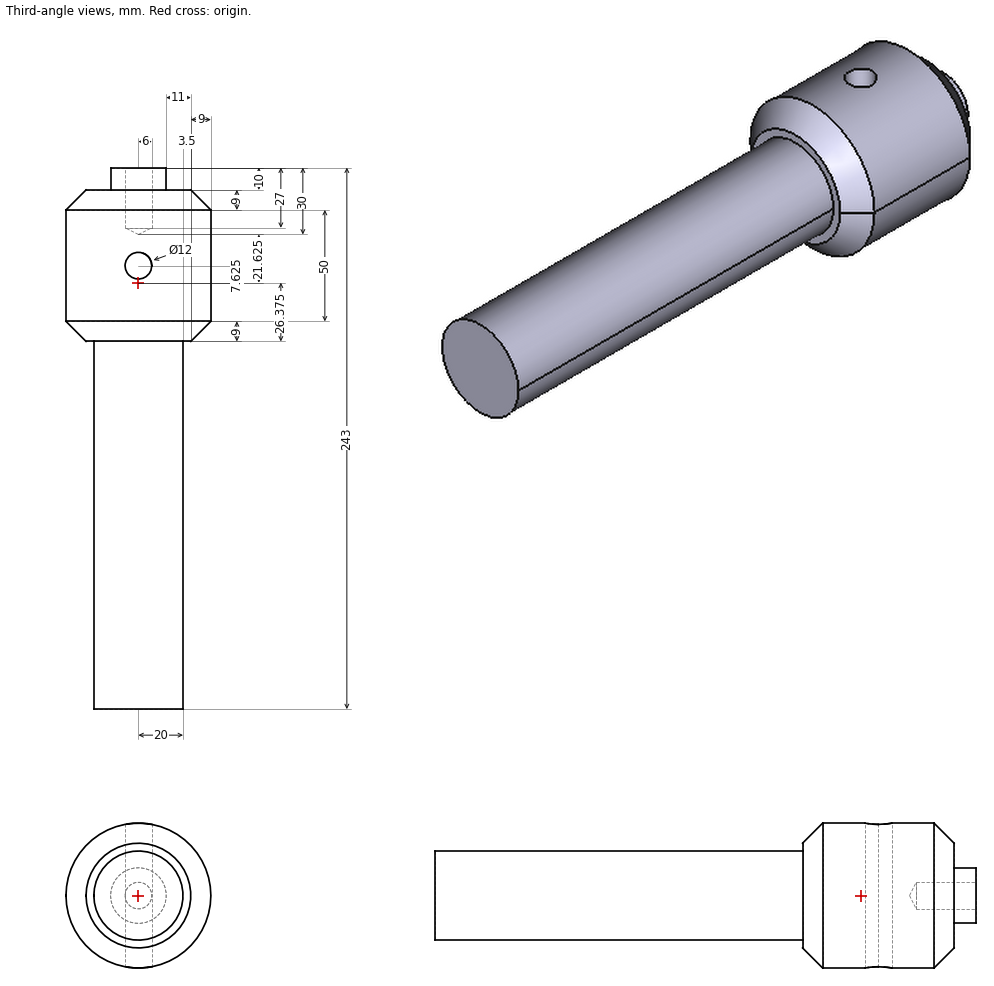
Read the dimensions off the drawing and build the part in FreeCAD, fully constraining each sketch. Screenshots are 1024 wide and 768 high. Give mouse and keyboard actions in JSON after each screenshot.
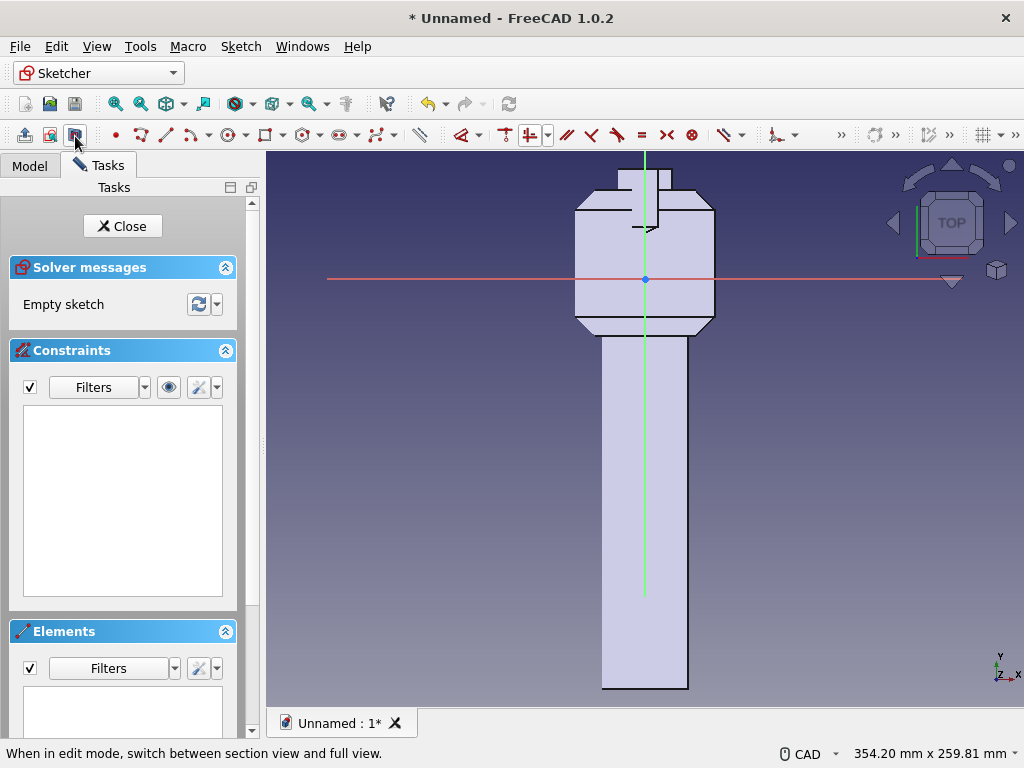
{"action": "scroll", "coordinate": [652, 249], "scroll_direction": "up", "scroll_amount": 12}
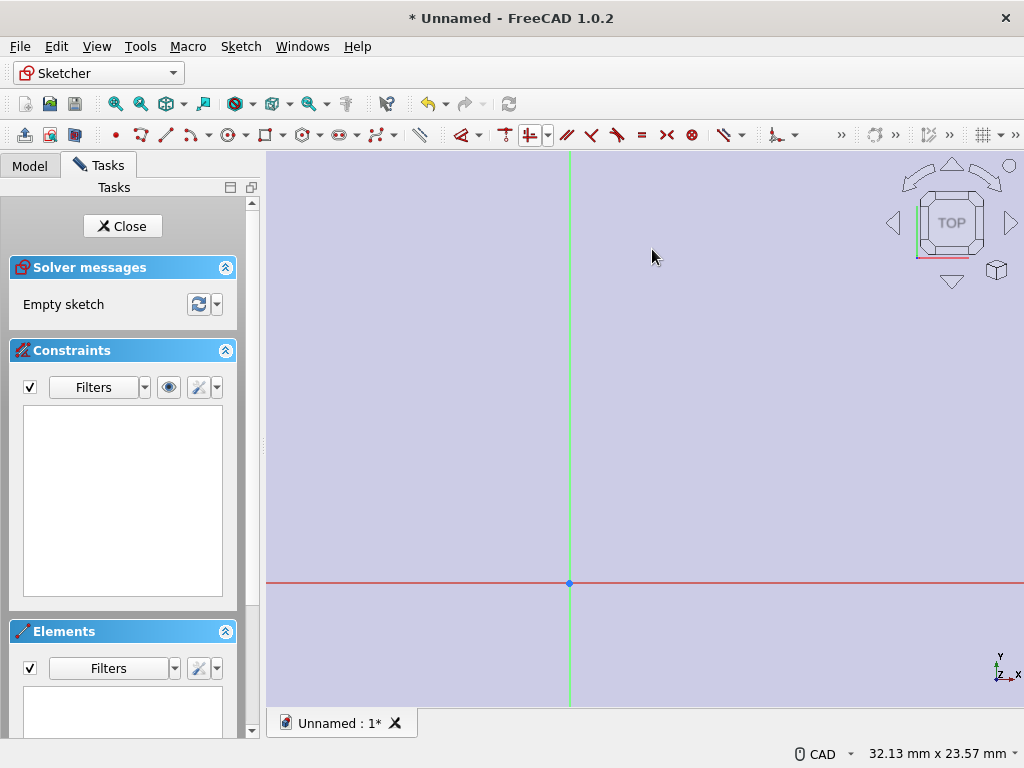
{"action": "left_click", "coordinate": [228, 136]}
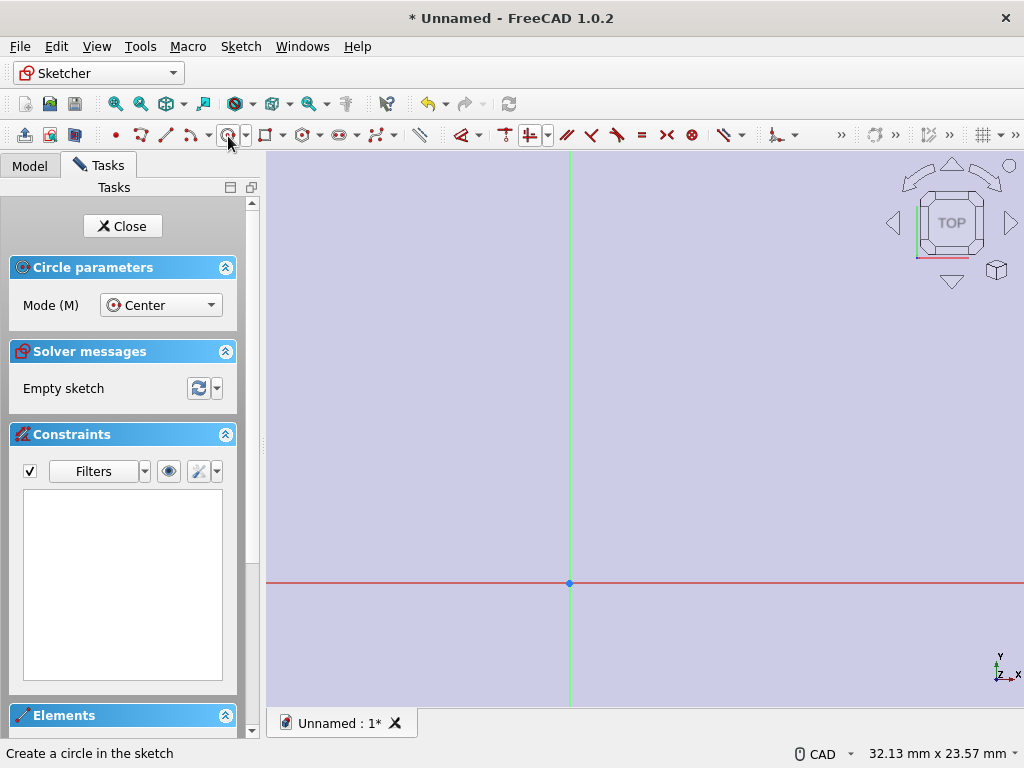
{"action": "left_click", "coordinate": [570, 403]}
{"action": "mouse_move", "coordinate": [670, 303]}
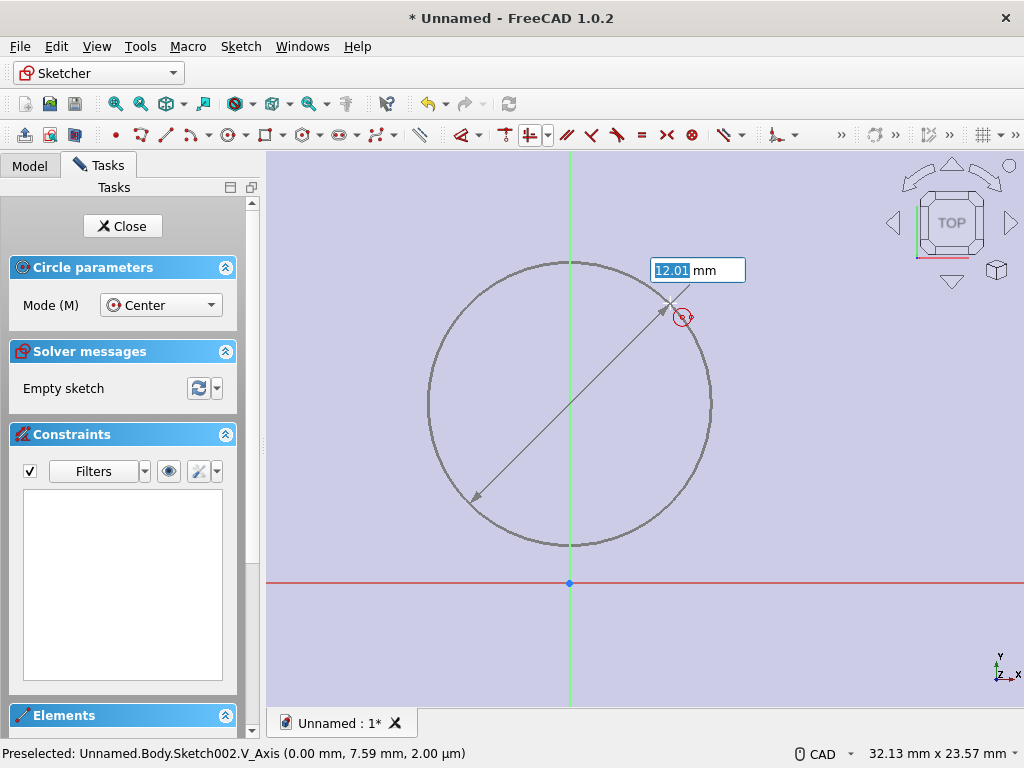
{"action": "type", "text": "12"}
{"action": "key", "text": "Return"}
{"action": "key", "text": "Escape"}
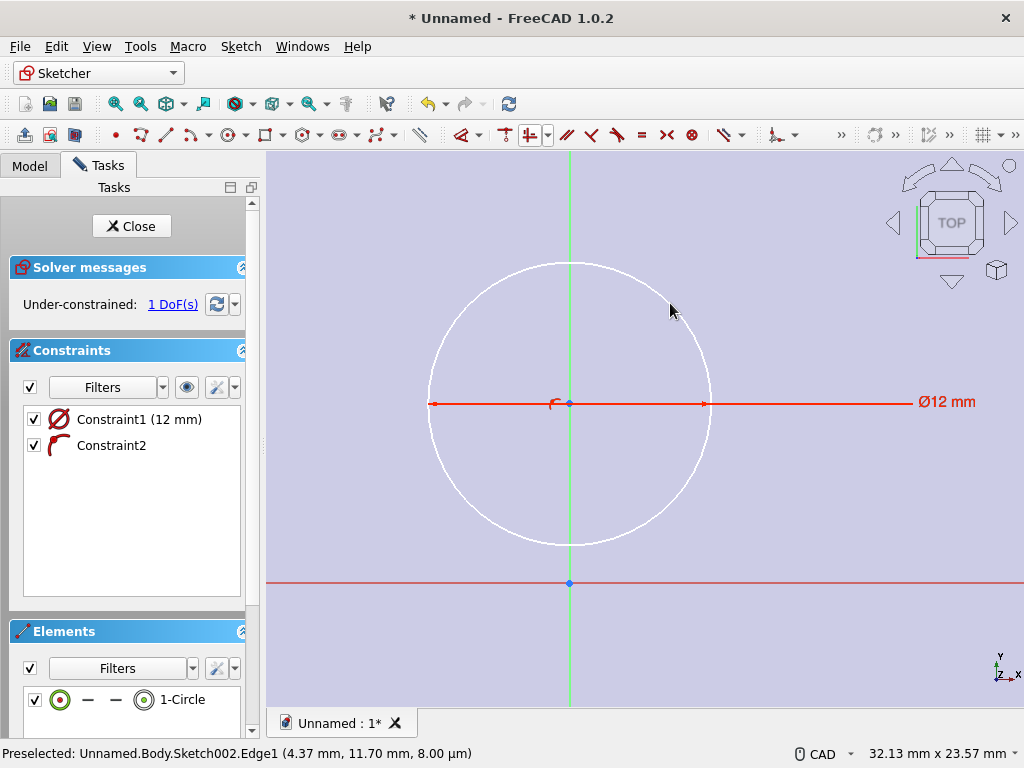
{"action": "left_click", "coordinate": [460, 136]}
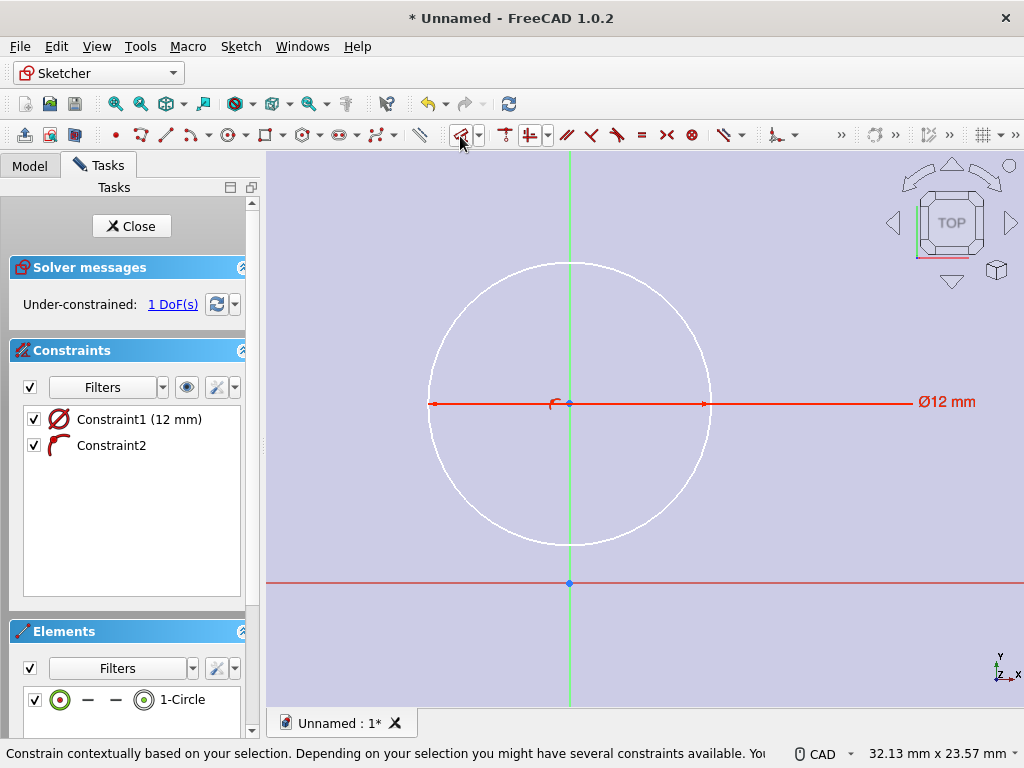
{"action": "left_click", "coordinate": [570, 404]}
{"action": "left_click", "coordinate": [604, 494]}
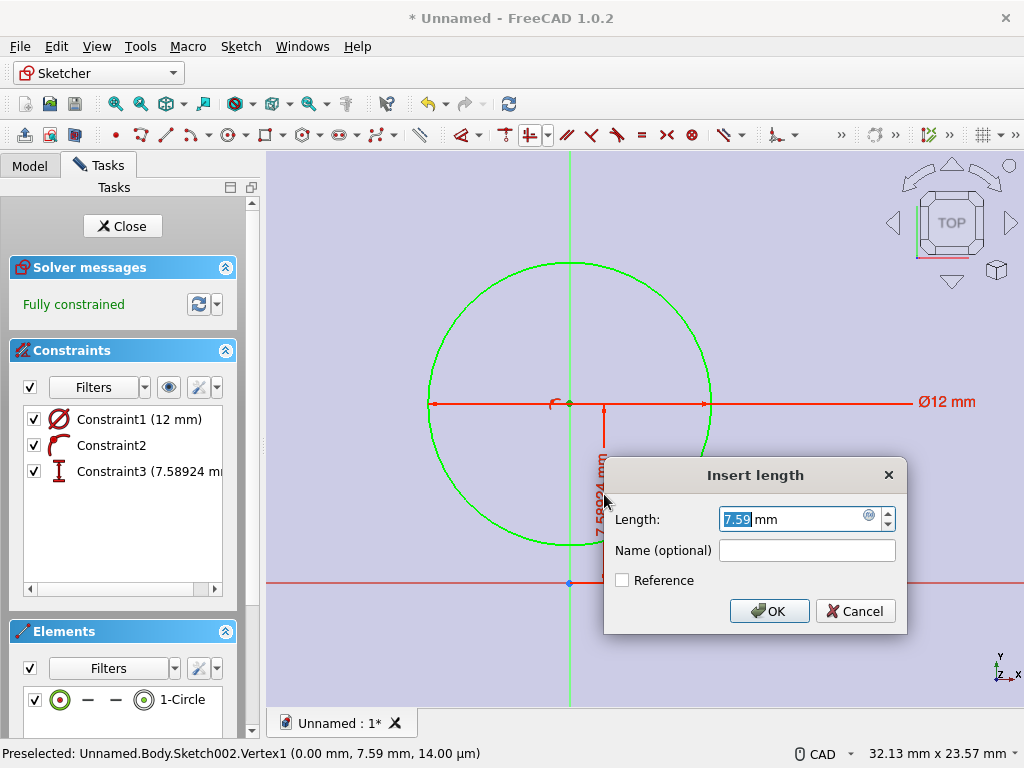
{"action": "type", "text": "7.625"}
{"action": "key", "text": "Return"}
{"action": "key", "text": "Escape"}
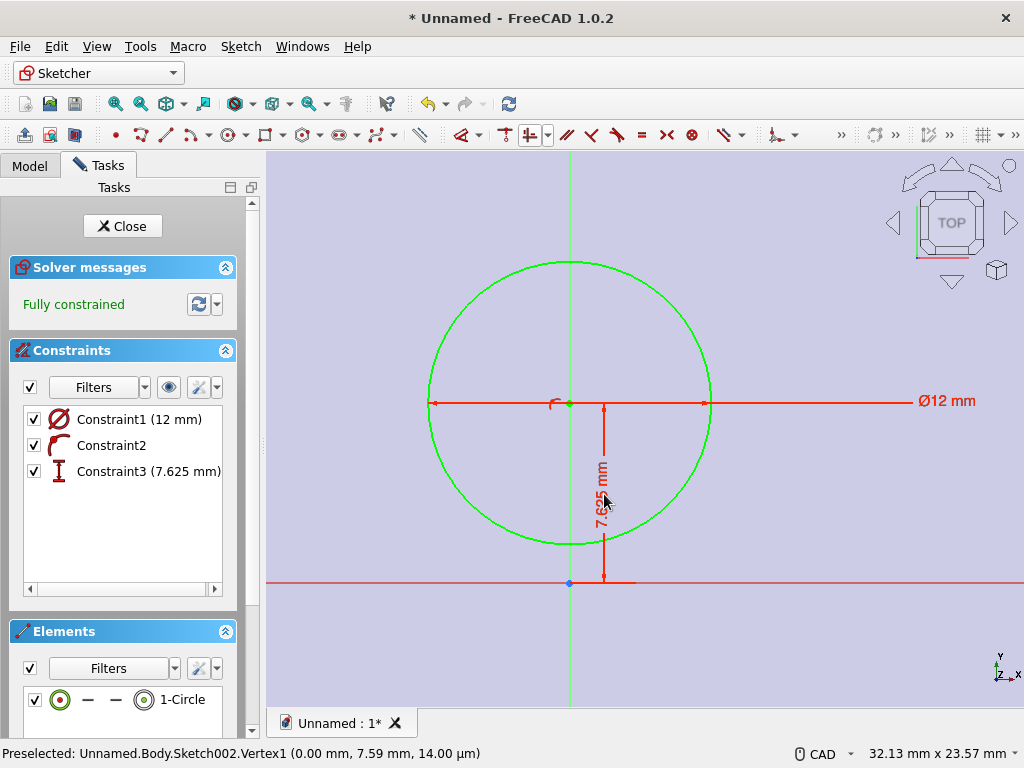
{"action": "left_click", "coordinate": [123, 226]}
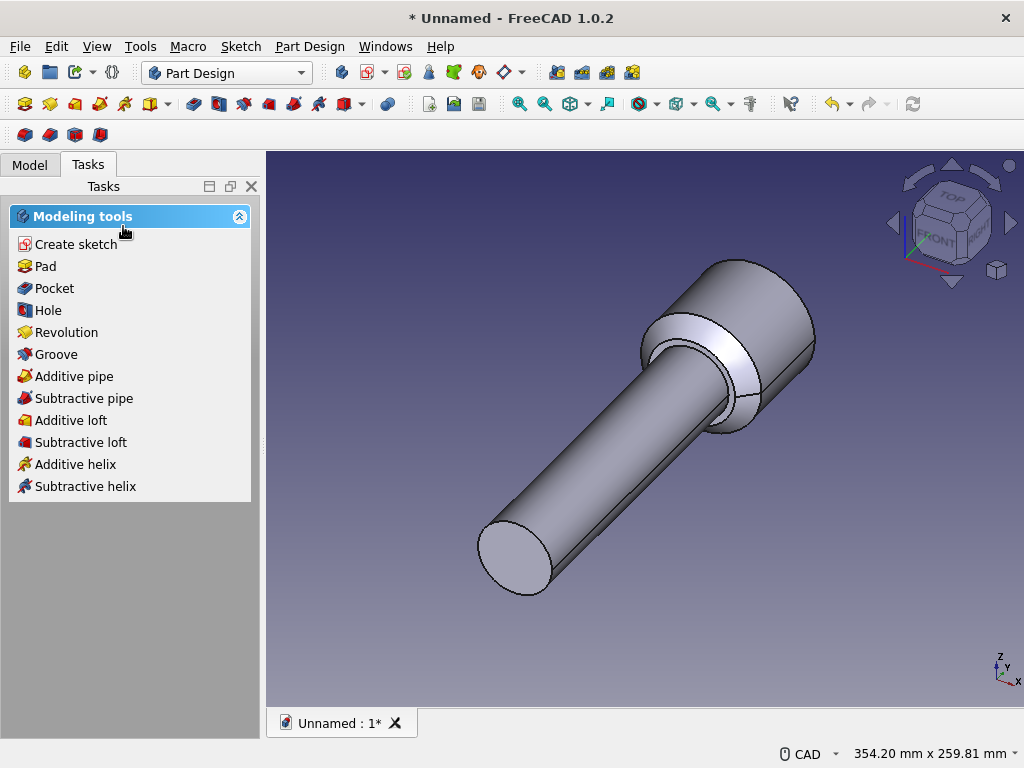
{"action": "left_click", "coordinate": [194, 104]}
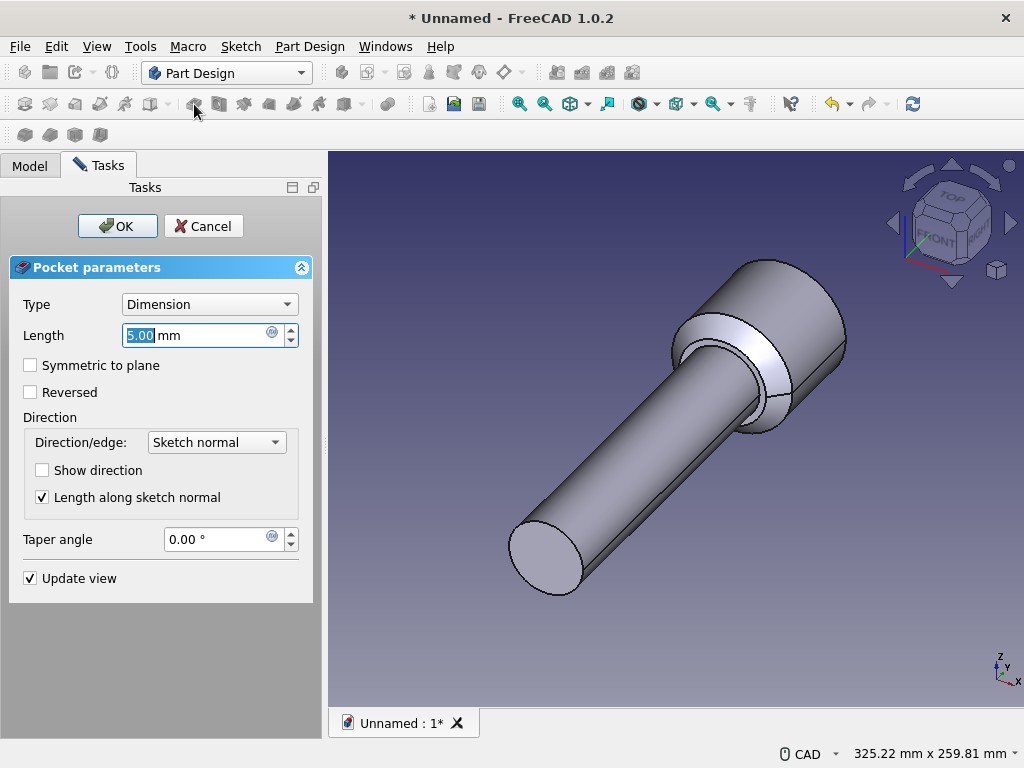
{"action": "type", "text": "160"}
{"action": "key", "text": "Tab"}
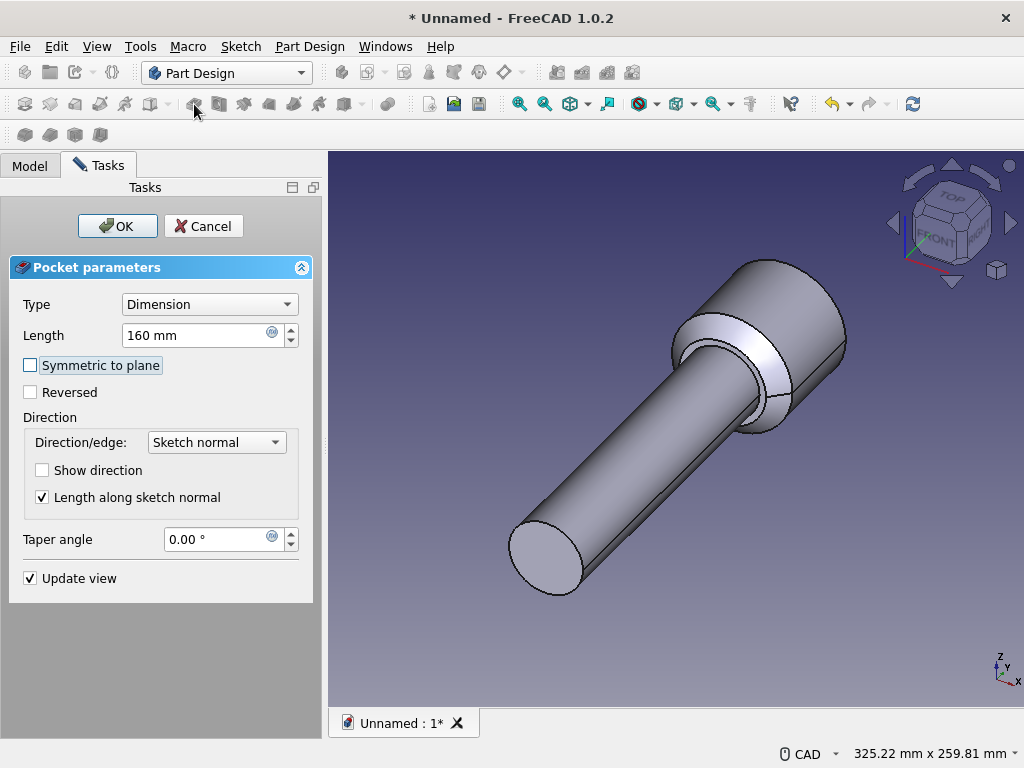
{"action": "left_click", "coordinate": [31, 365]}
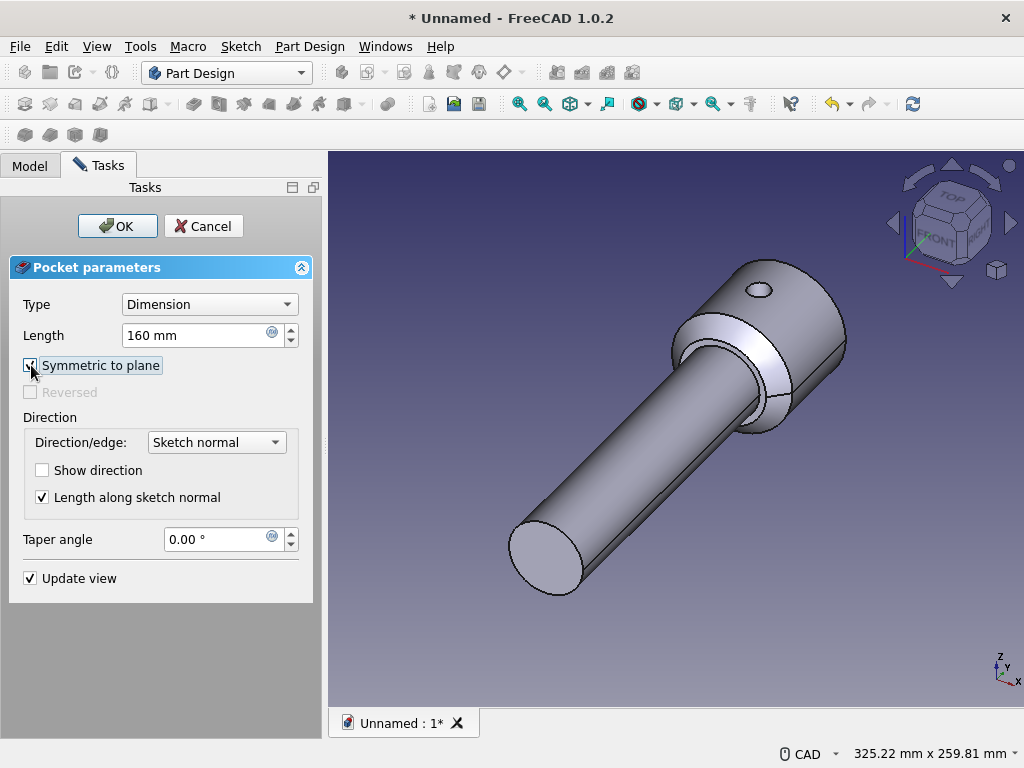
{"action": "left_click", "coordinate": [118, 226]}